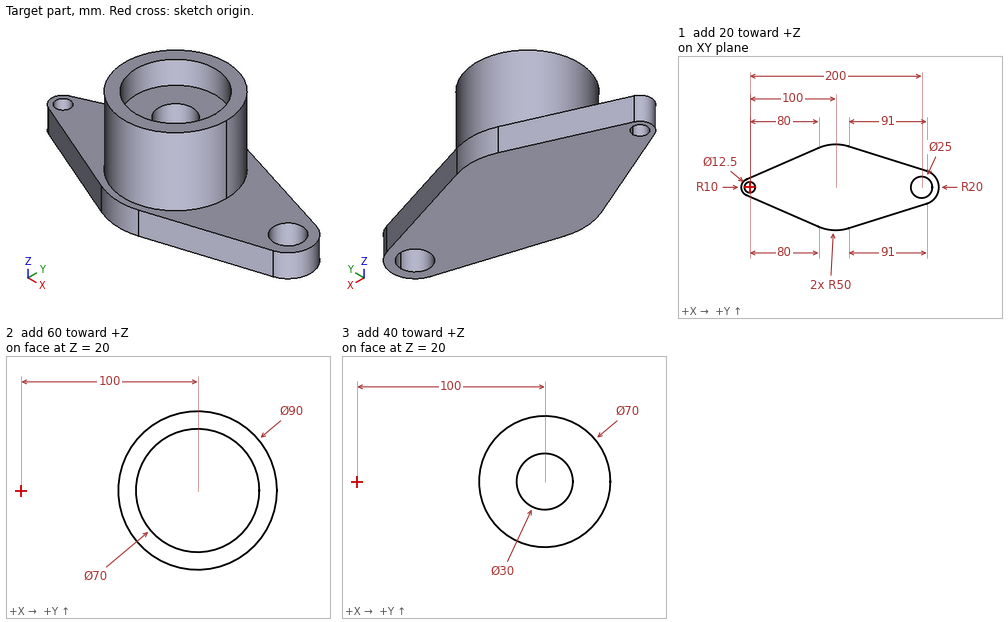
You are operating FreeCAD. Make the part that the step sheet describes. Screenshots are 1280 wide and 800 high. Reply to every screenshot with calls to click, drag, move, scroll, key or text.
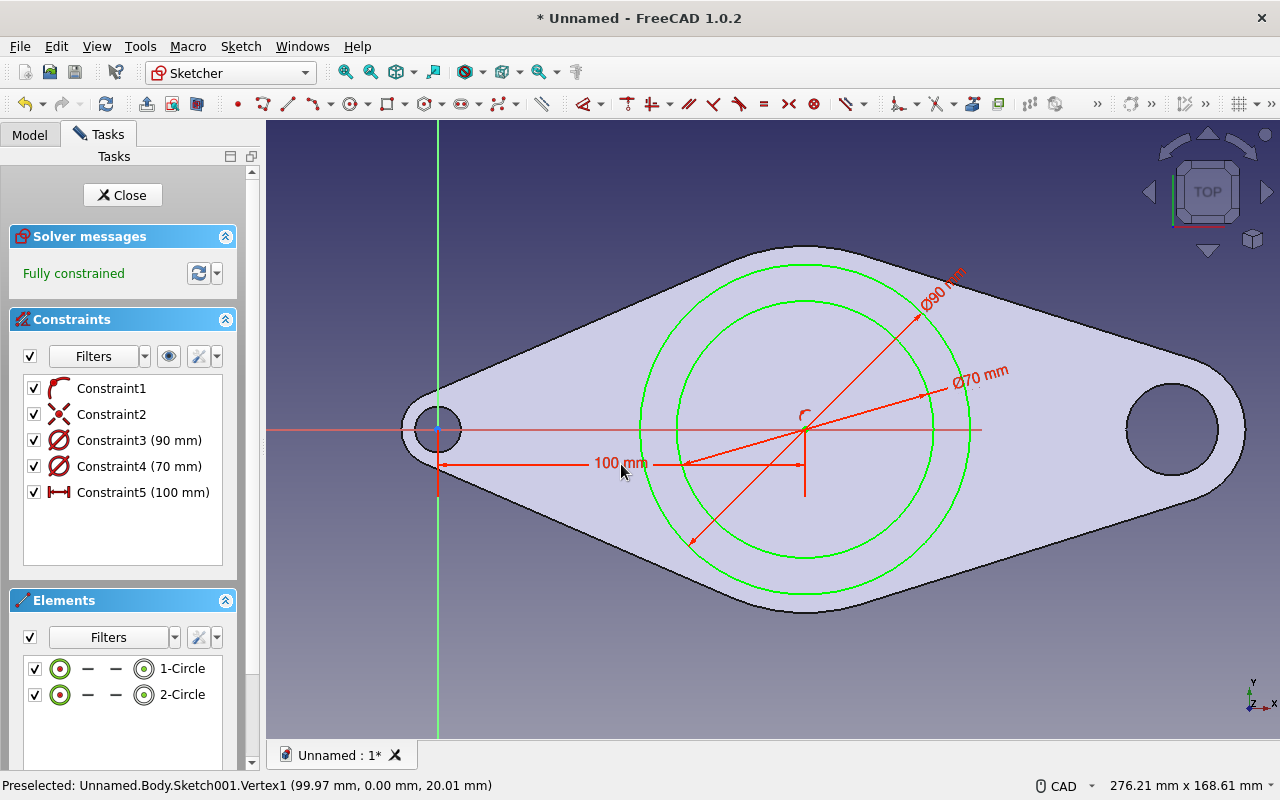
click(123, 195)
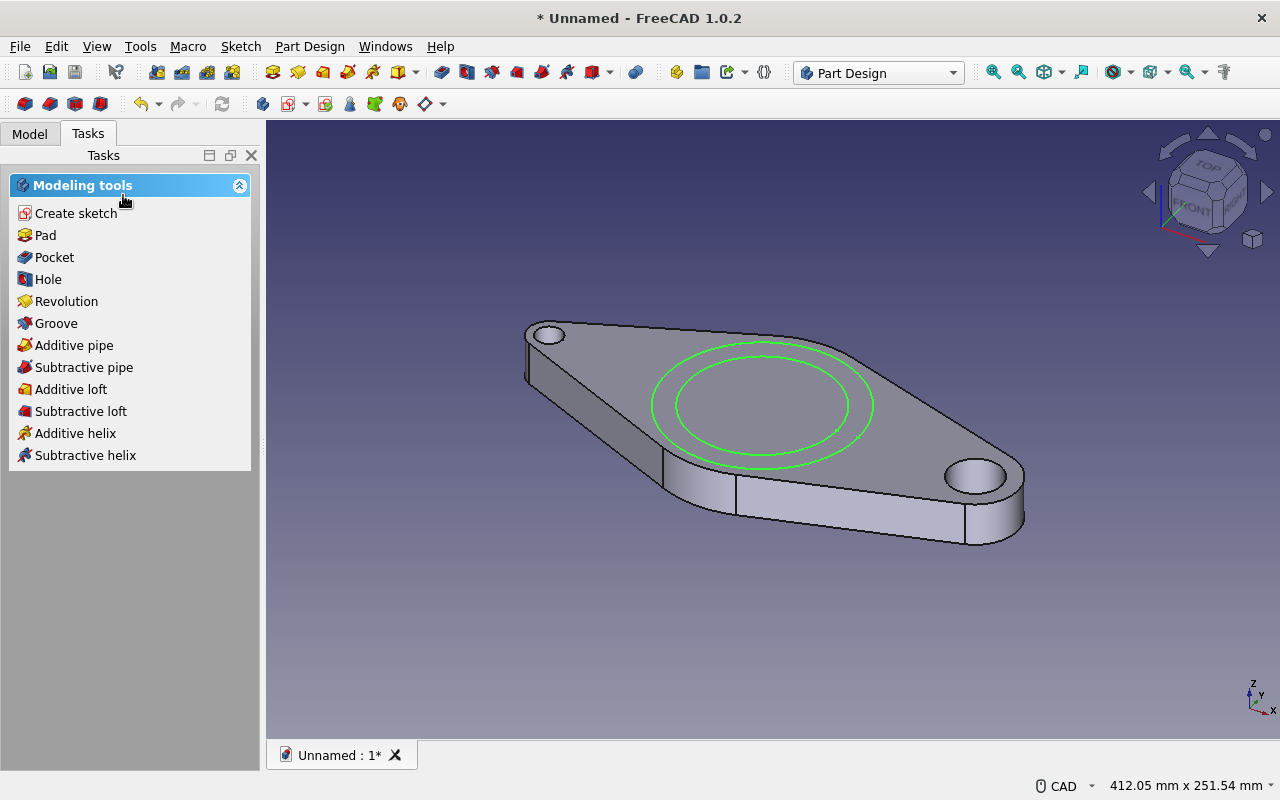
click(273, 72)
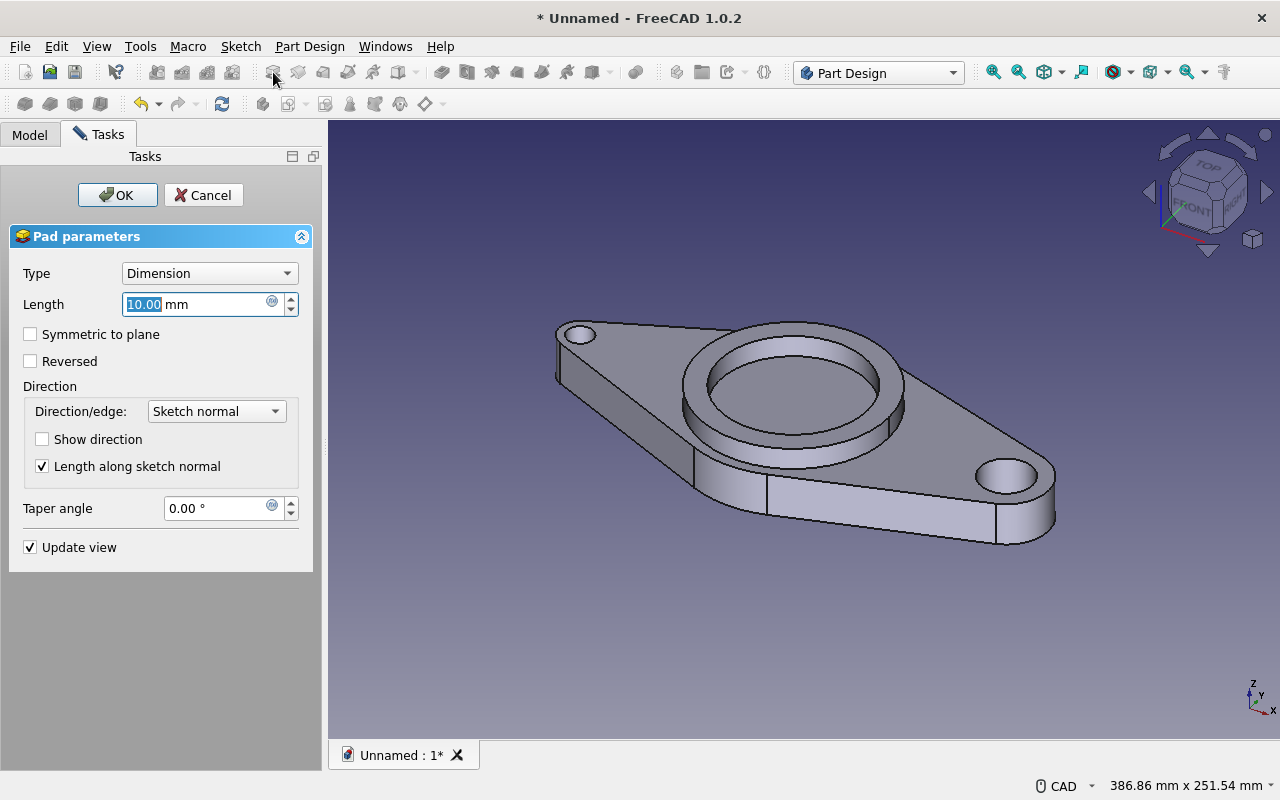
text(60)
key(Tab)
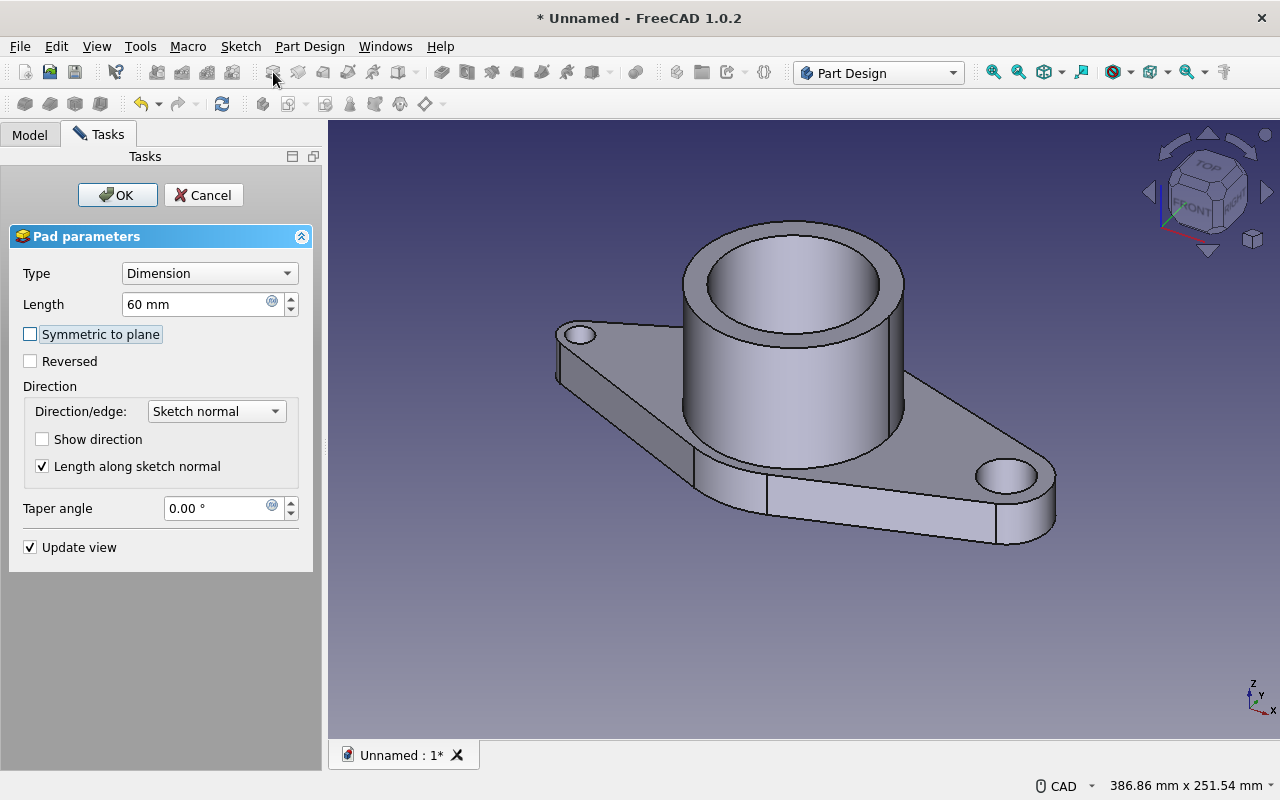
click(118, 195)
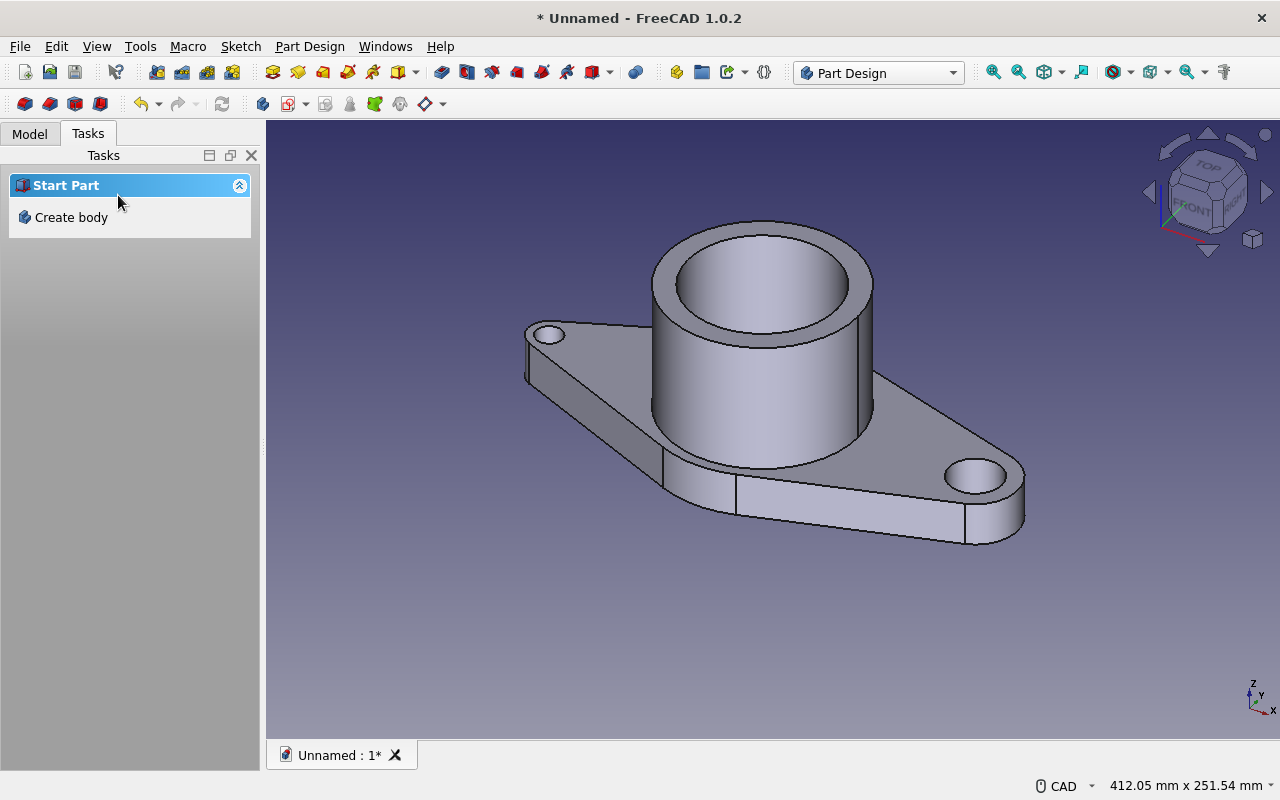
click(913, 454)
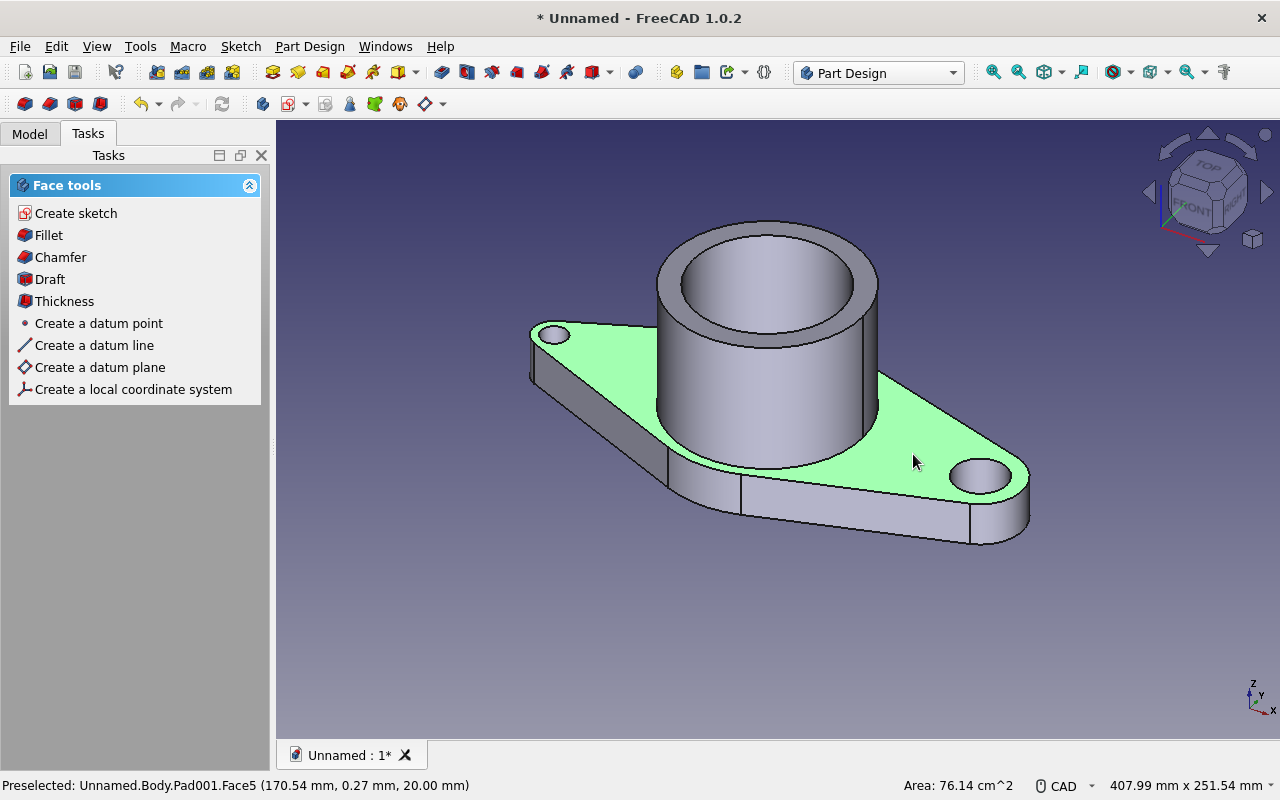
click(288, 104)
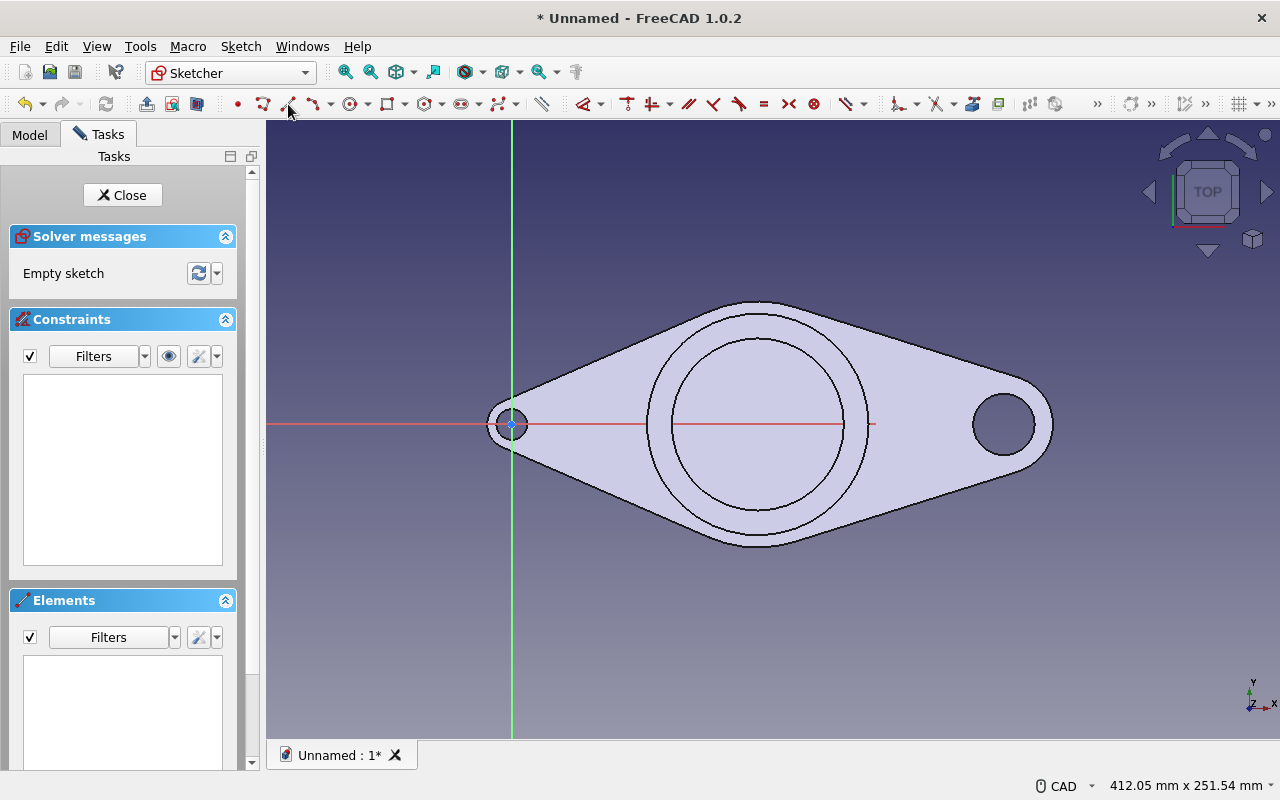
click(197, 104)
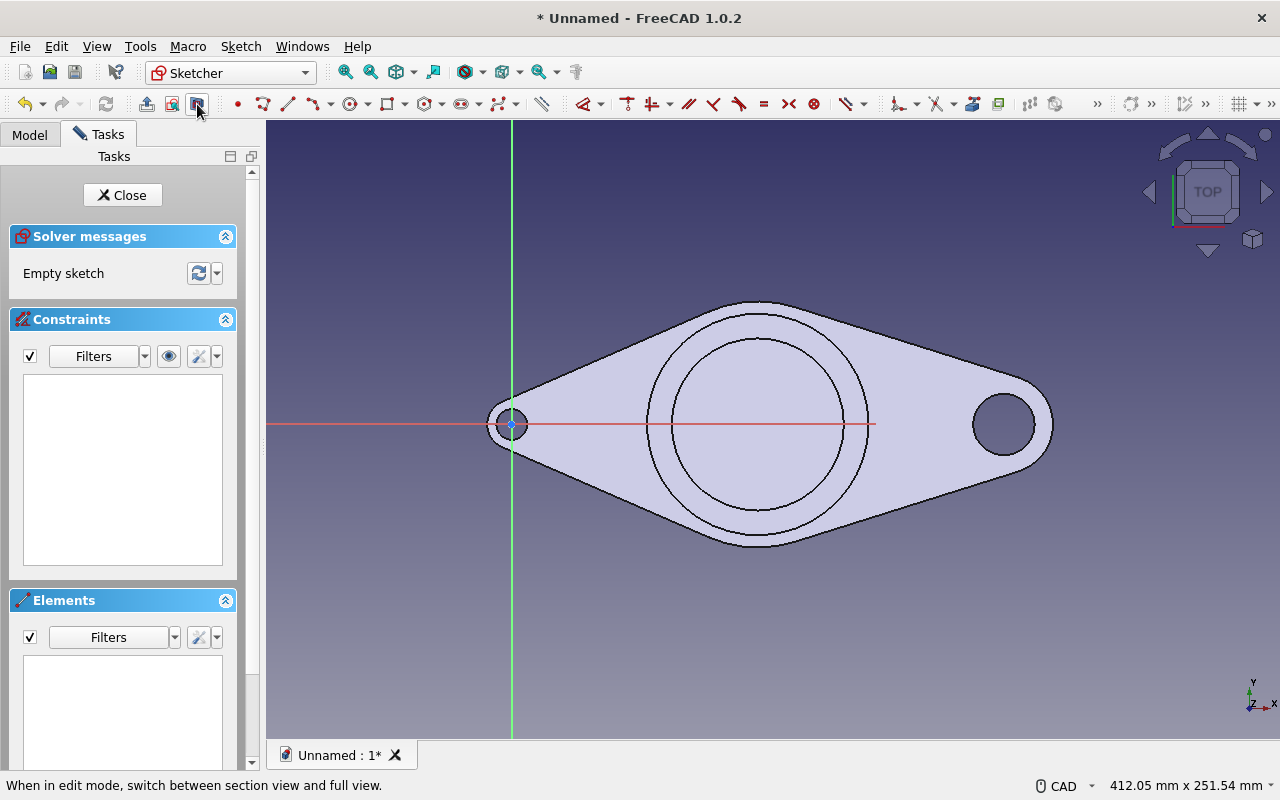
scroll(645, 418, up, 3)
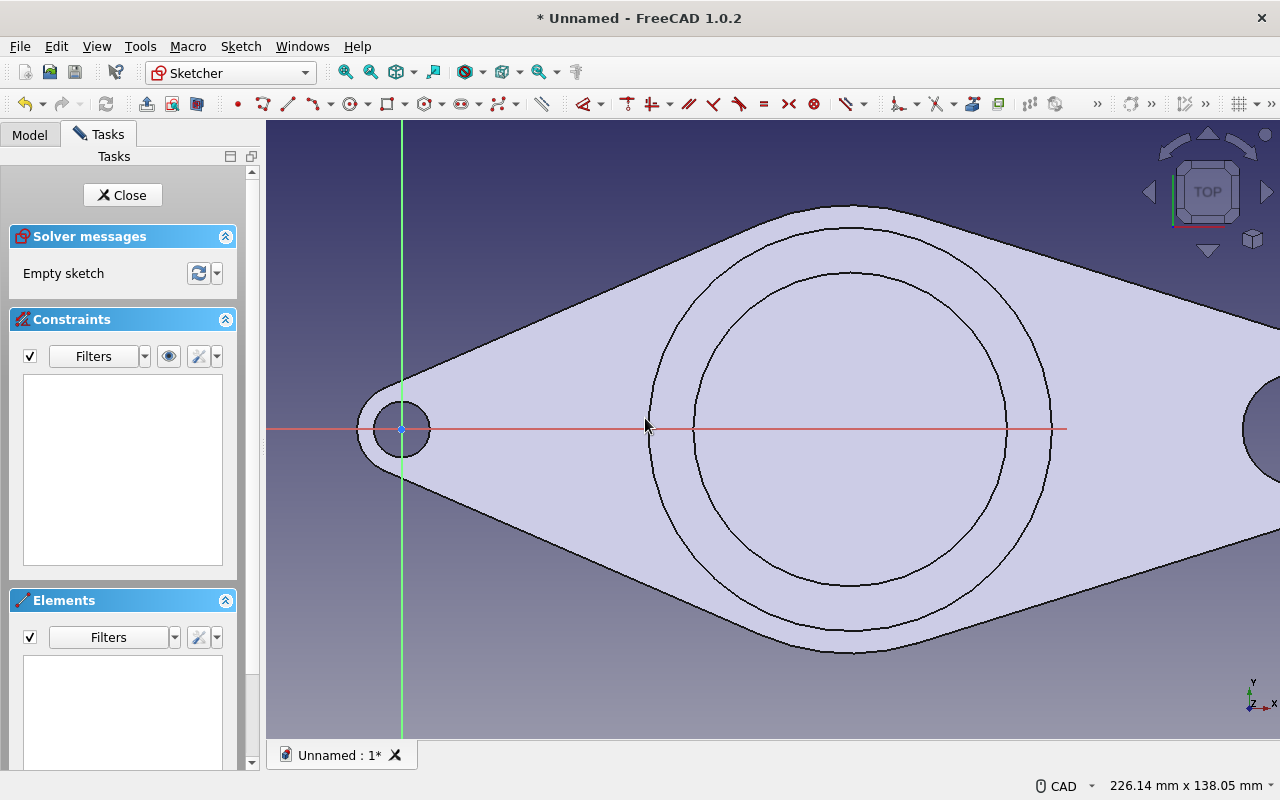
click(350, 104)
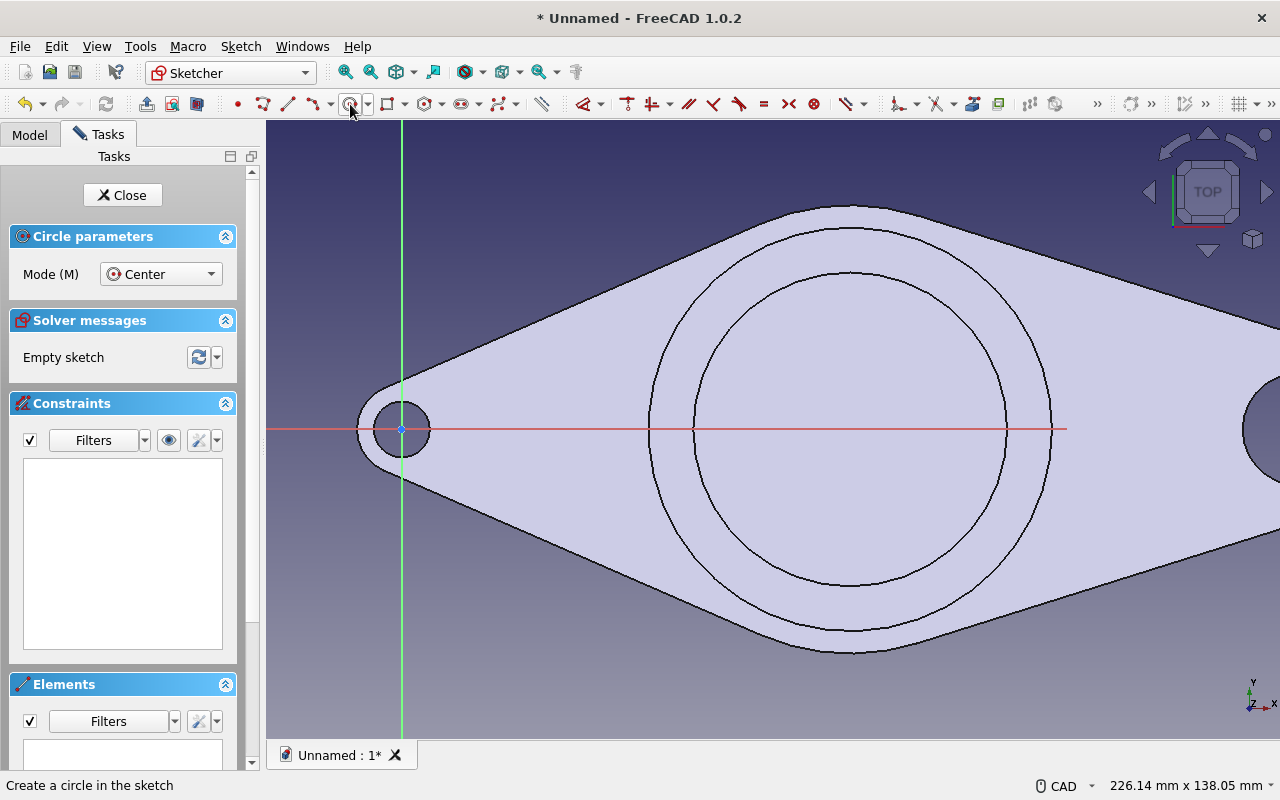
click(850, 429)
click(961, 318)